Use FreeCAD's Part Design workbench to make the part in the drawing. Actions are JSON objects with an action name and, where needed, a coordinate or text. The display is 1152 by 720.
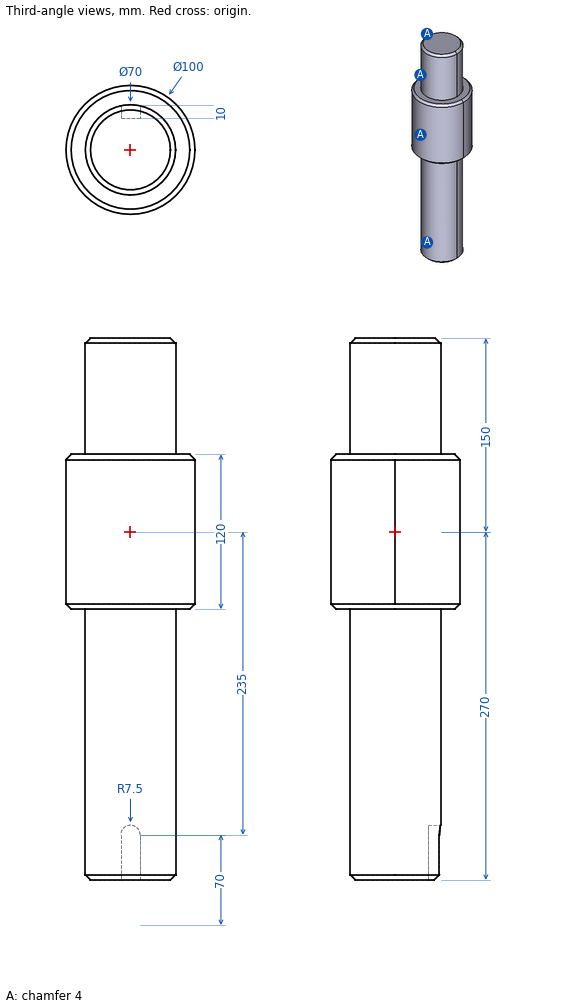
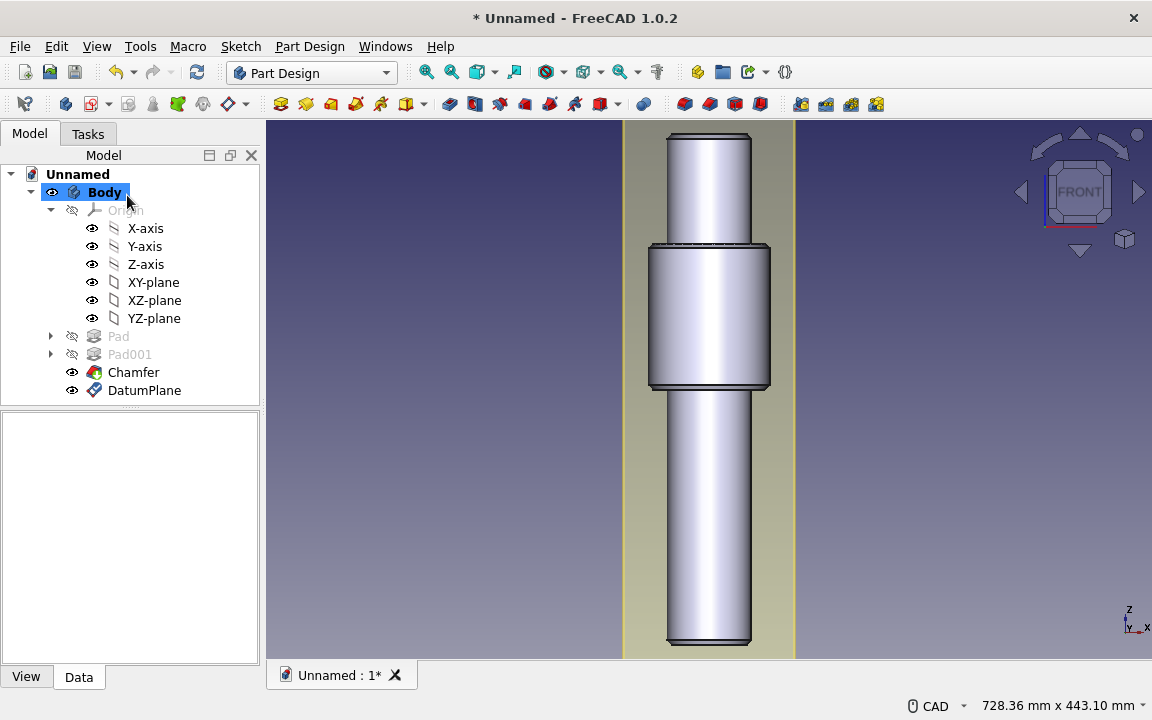
{"action": "left_click", "coordinate": [117, 390]}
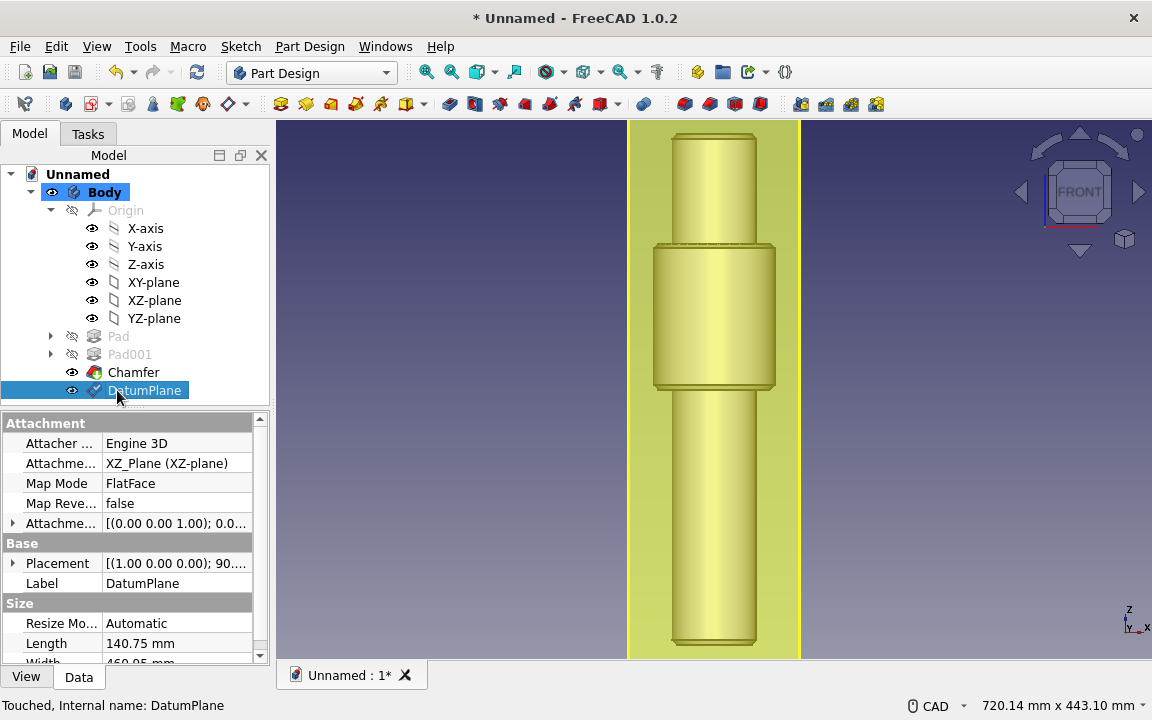
{"action": "left_click", "coordinate": [90, 104]}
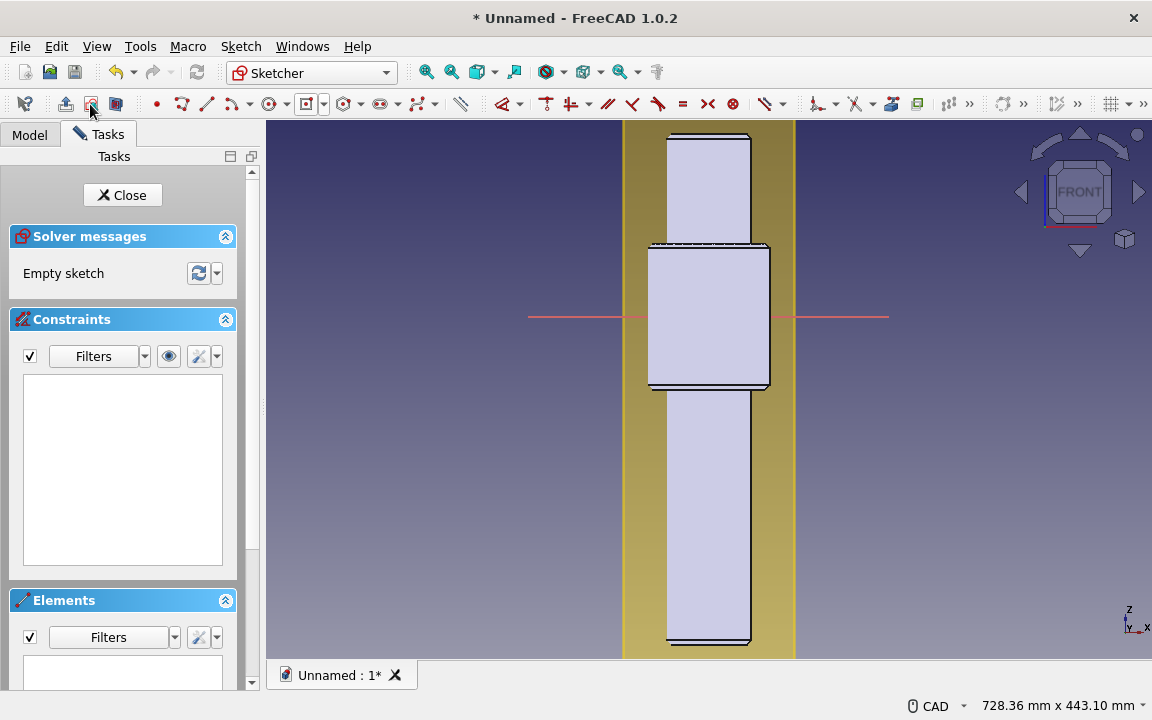
{"action": "key", "text": "q s"}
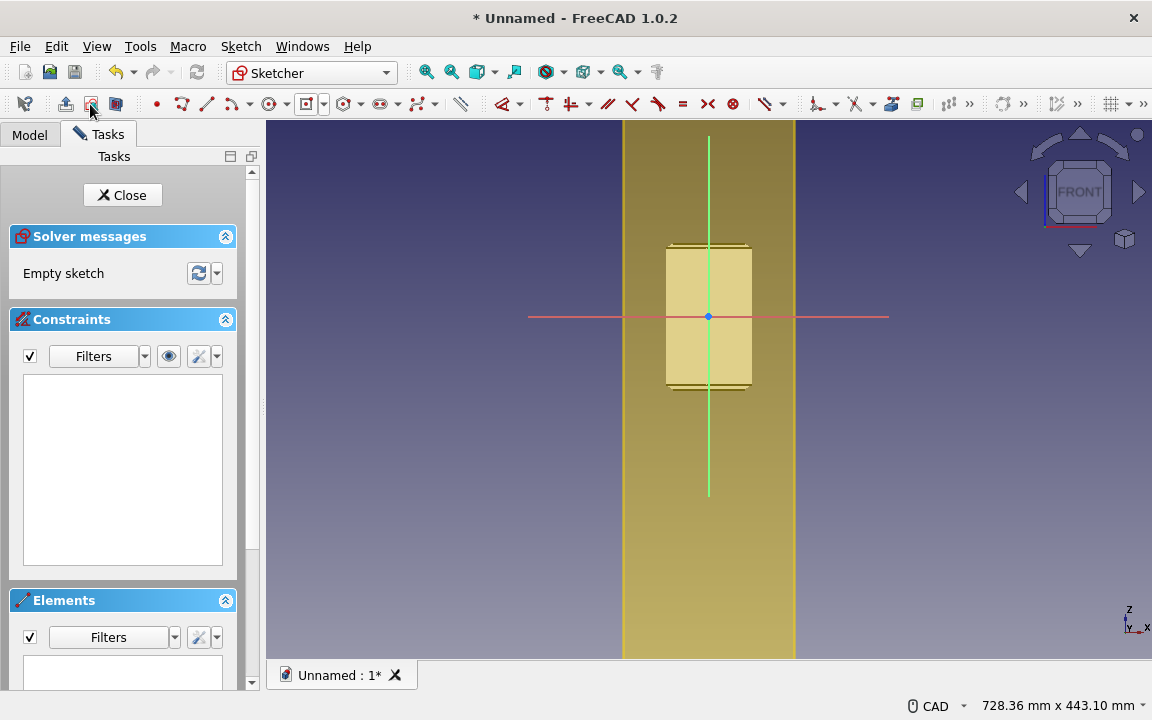
{"action": "scroll", "coordinate": [640, 390], "scroll_direction": "down", "scroll_amount": 5}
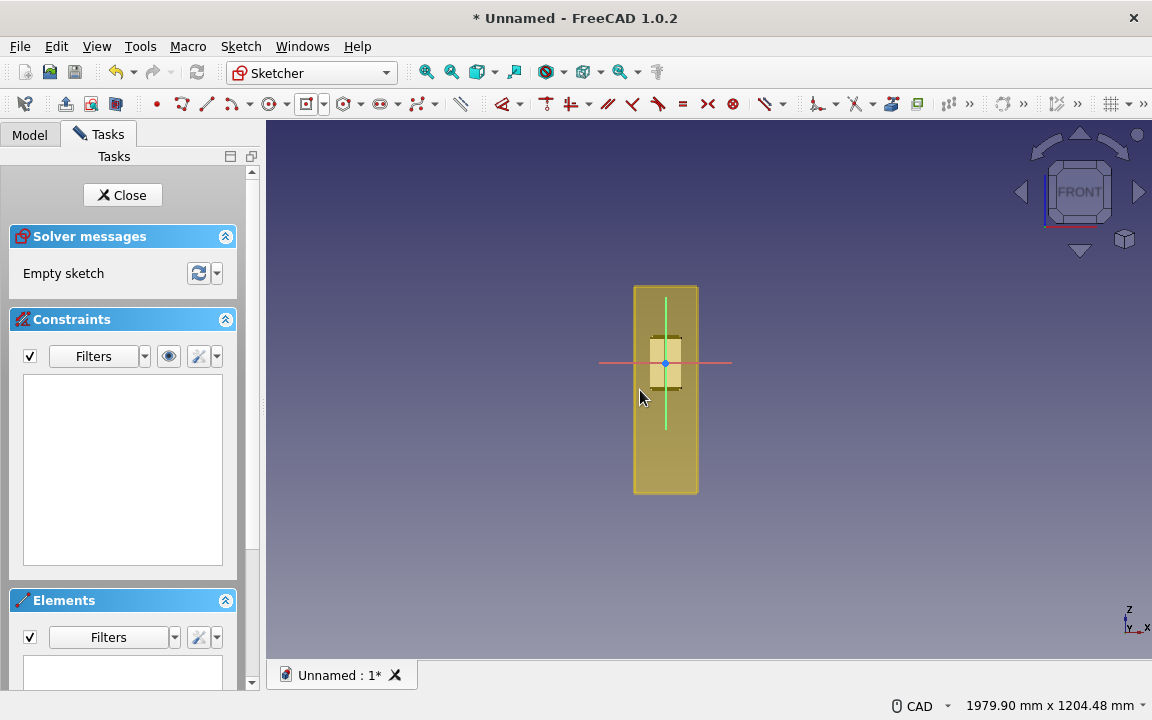
{"action": "scroll", "coordinate": [669, 494], "scroll_direction": "up", "scroll_amount": 11}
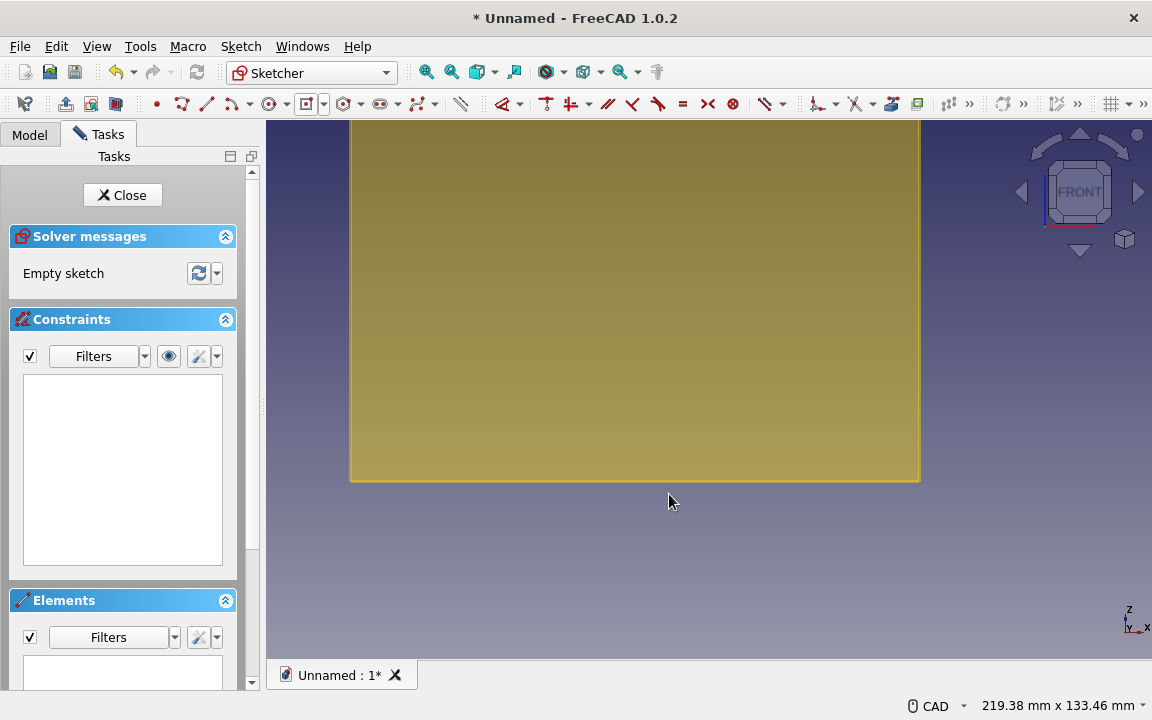
{"action": "key", "text": "g m"}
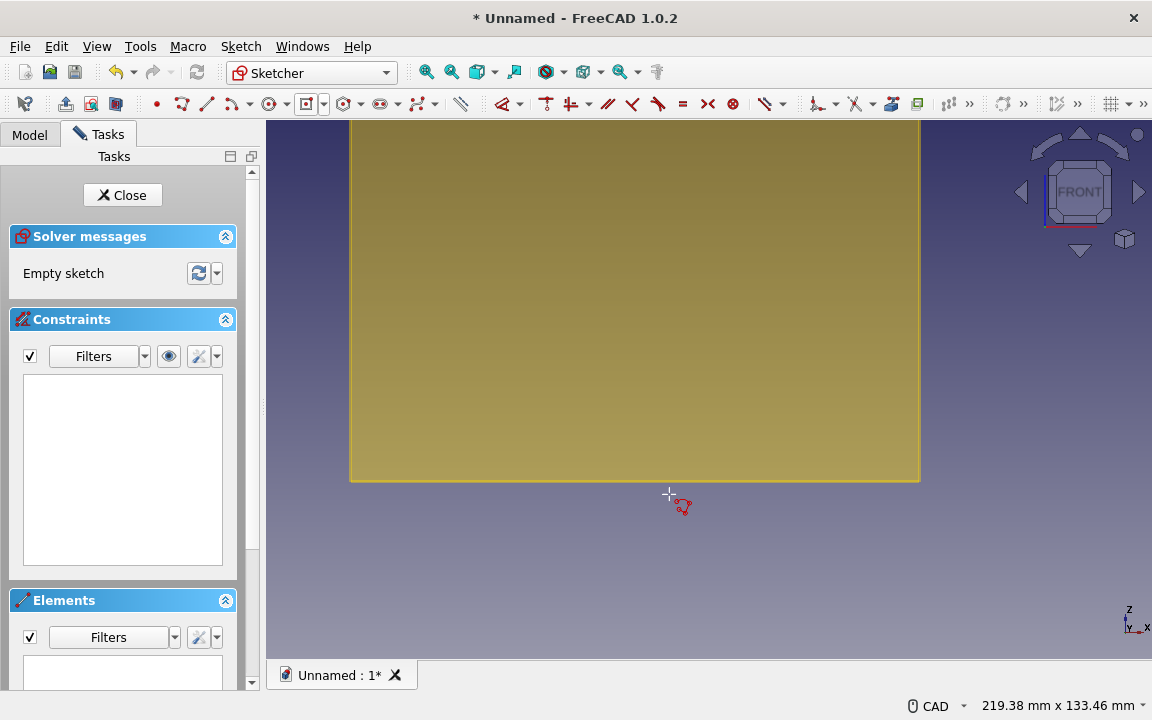
{"action": "left_click", "coordinate": [665, 258]}
{"action": "left_click", "coordinate": [665, 540]}
{"action": "left_click", "coordinate": [604, 540]}
{"action": "left_click", "coordinate": [604, 258]}
{"action": "right_click", "coordinate": [604, 258]}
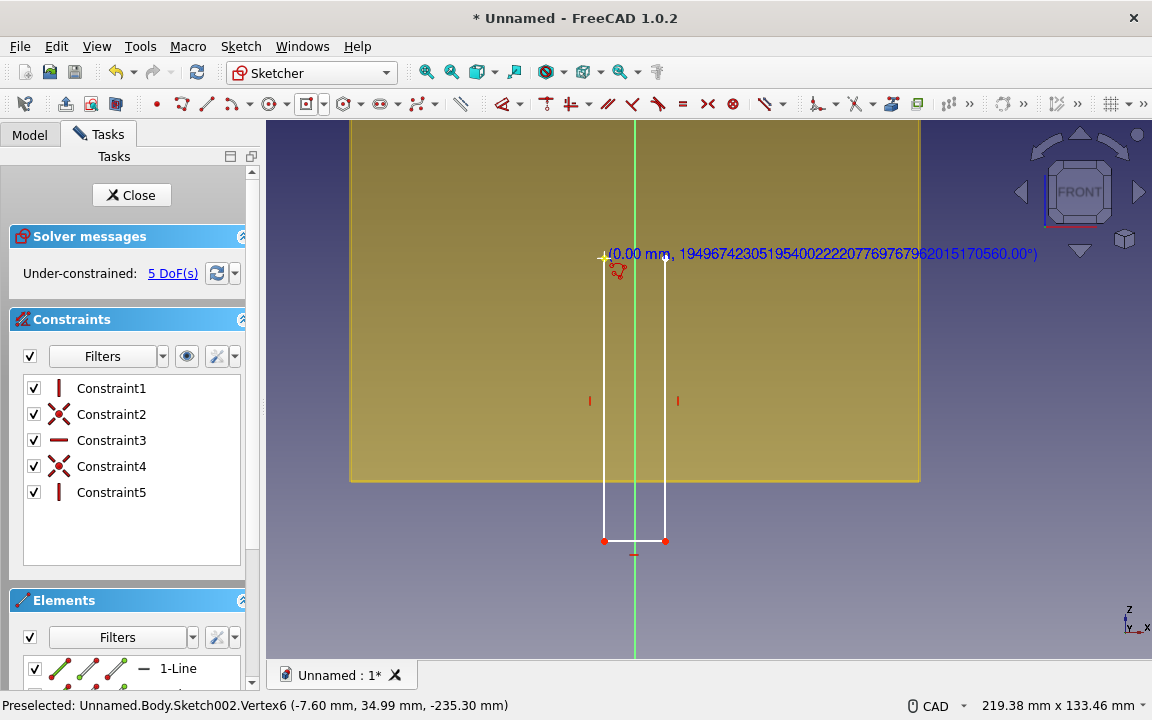
{"action": "key", "text": "g 3 a"}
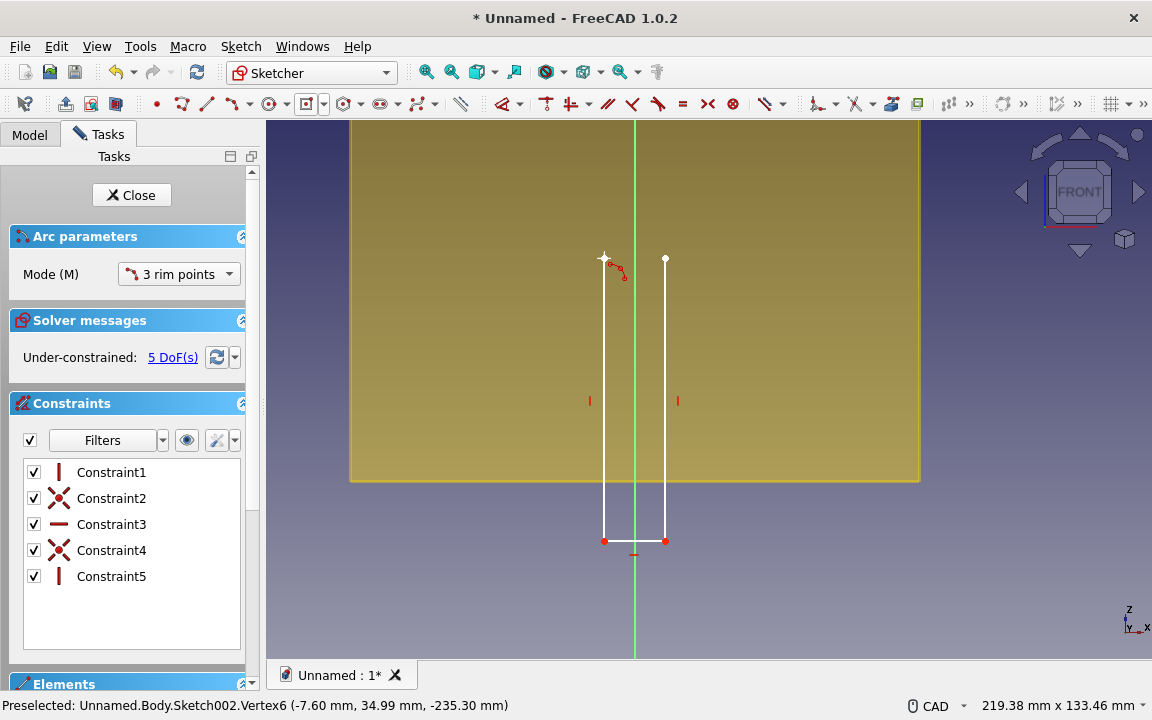
{"action": "left_click", "coordinate": [604, 259]}
{"action": "left_click", "coordinate": [665, 259]}
{"action": "left_click", "coordinate": [653, 233]}
{"action": "key", "text": "Escape"}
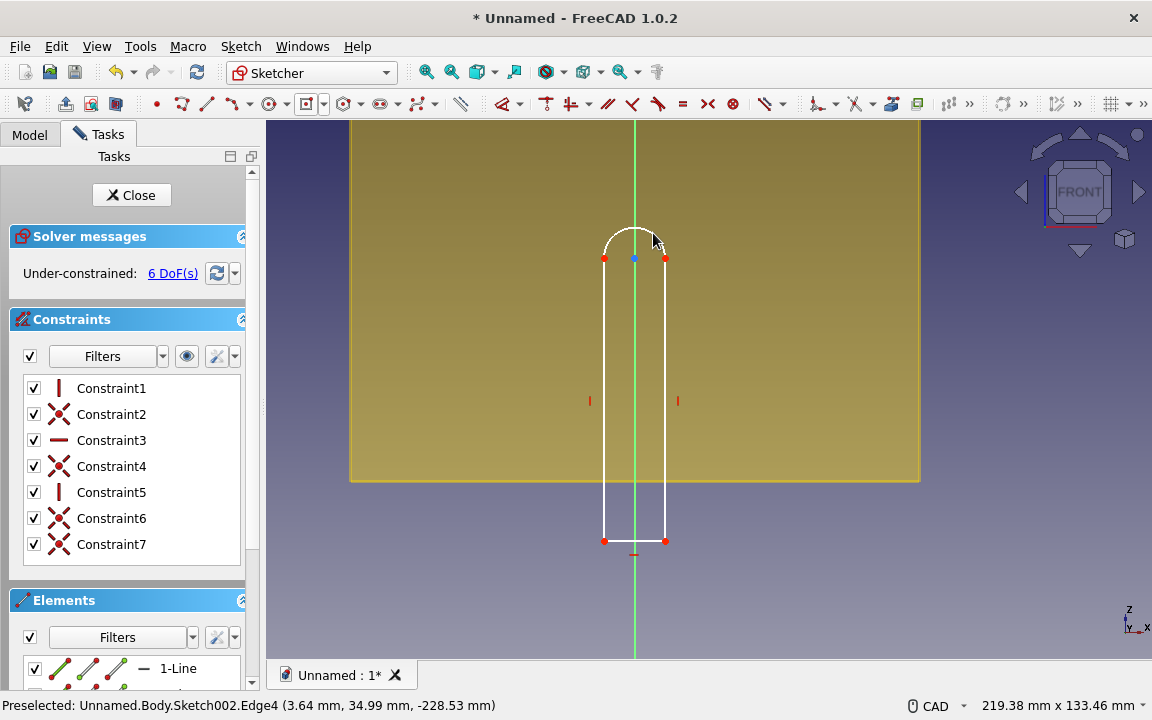
{"action": "left_click", "coordinate": [665, 344]}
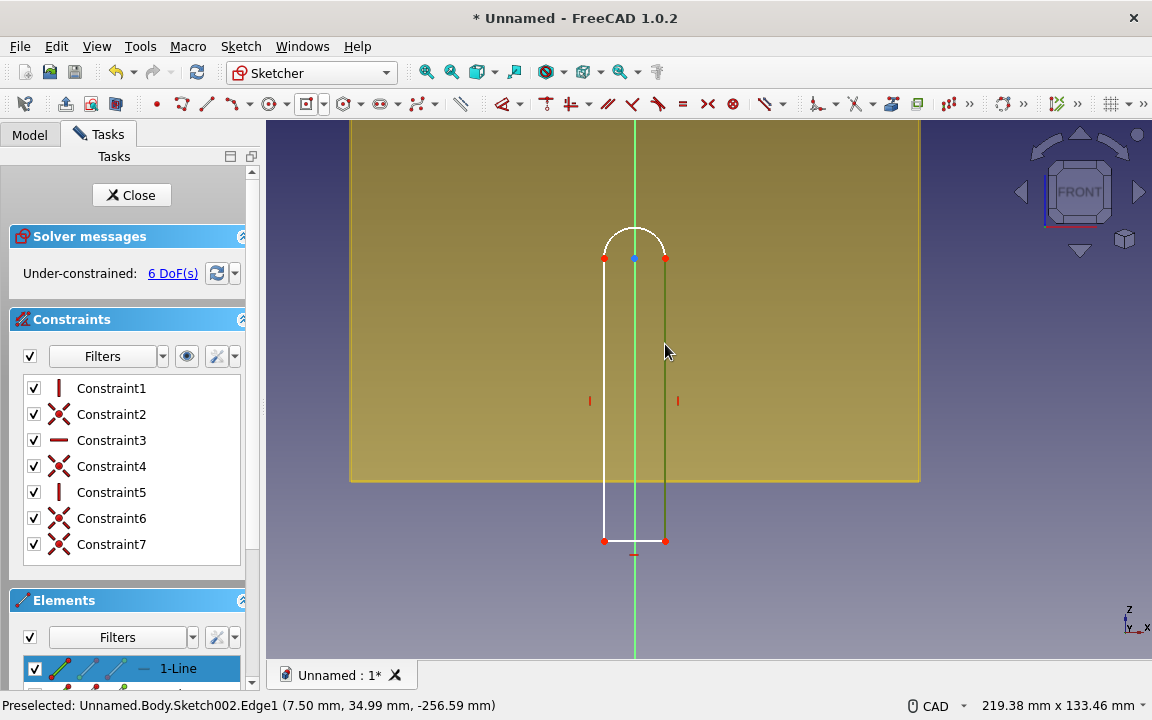
{"action": "left_click", "coordinate": [653, 234]}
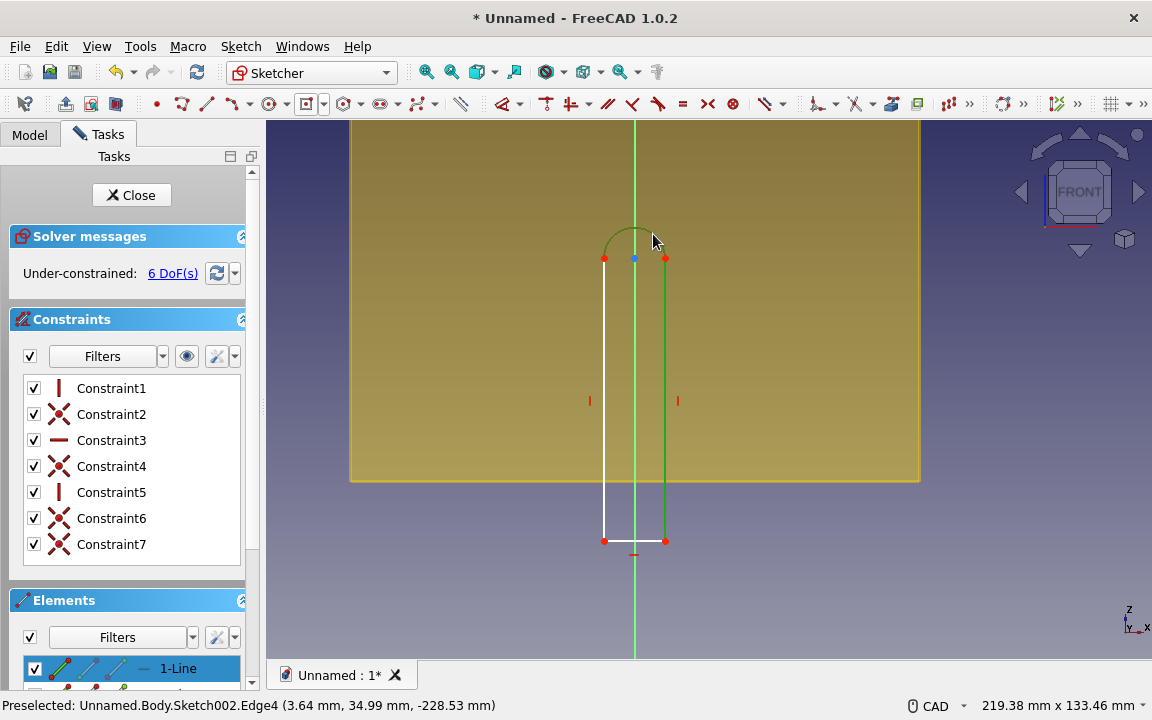
{"action": "key", "text": "t"}